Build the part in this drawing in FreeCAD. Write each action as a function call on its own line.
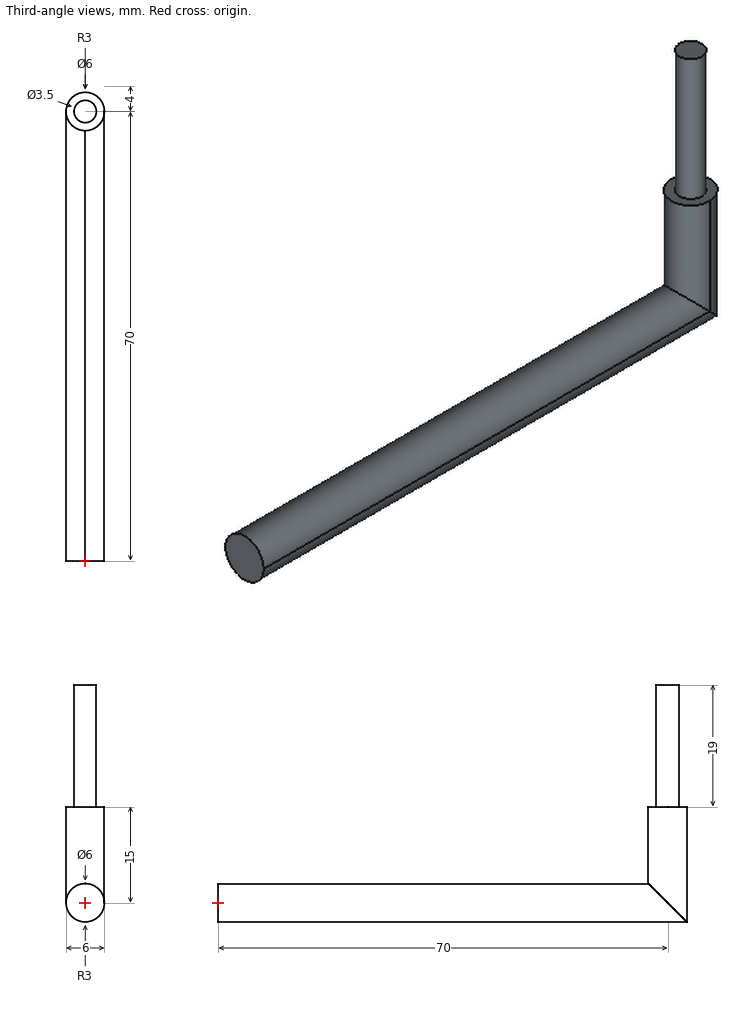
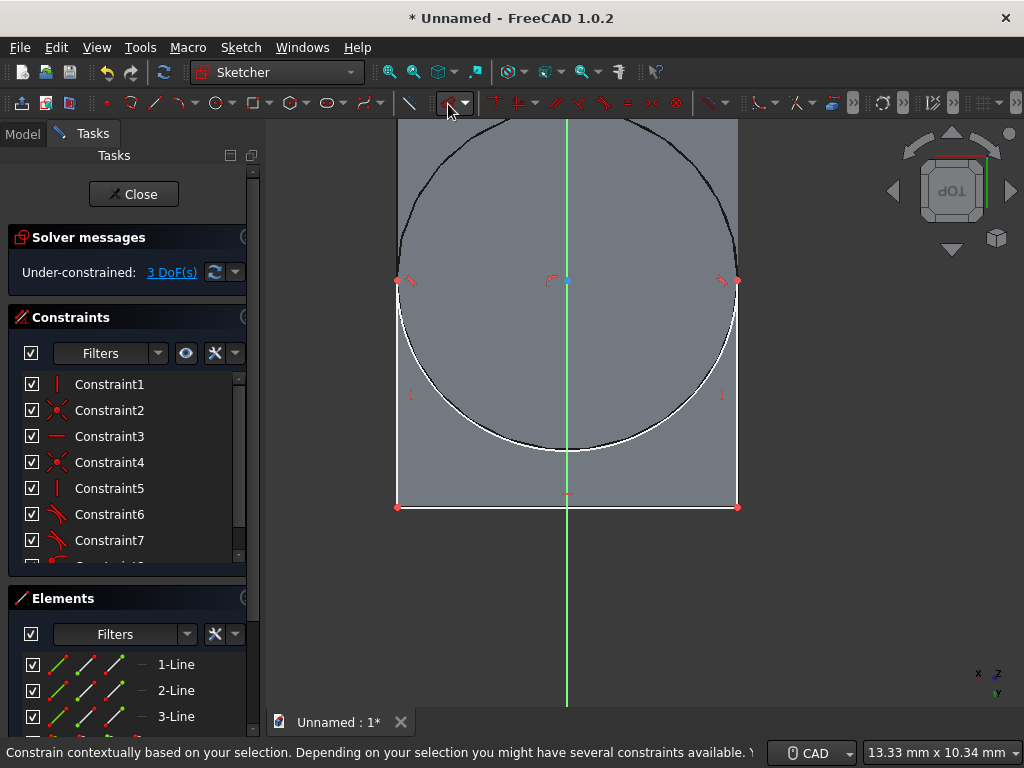
click(467, 419)
click(448, 445)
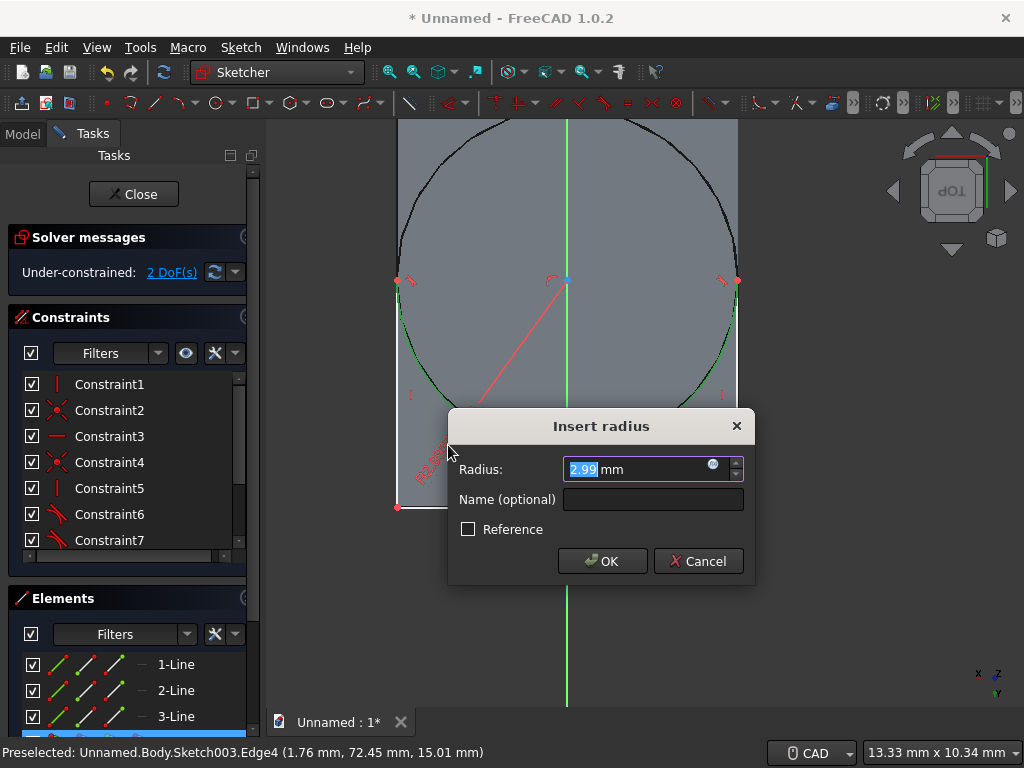
text(3)
key(Return)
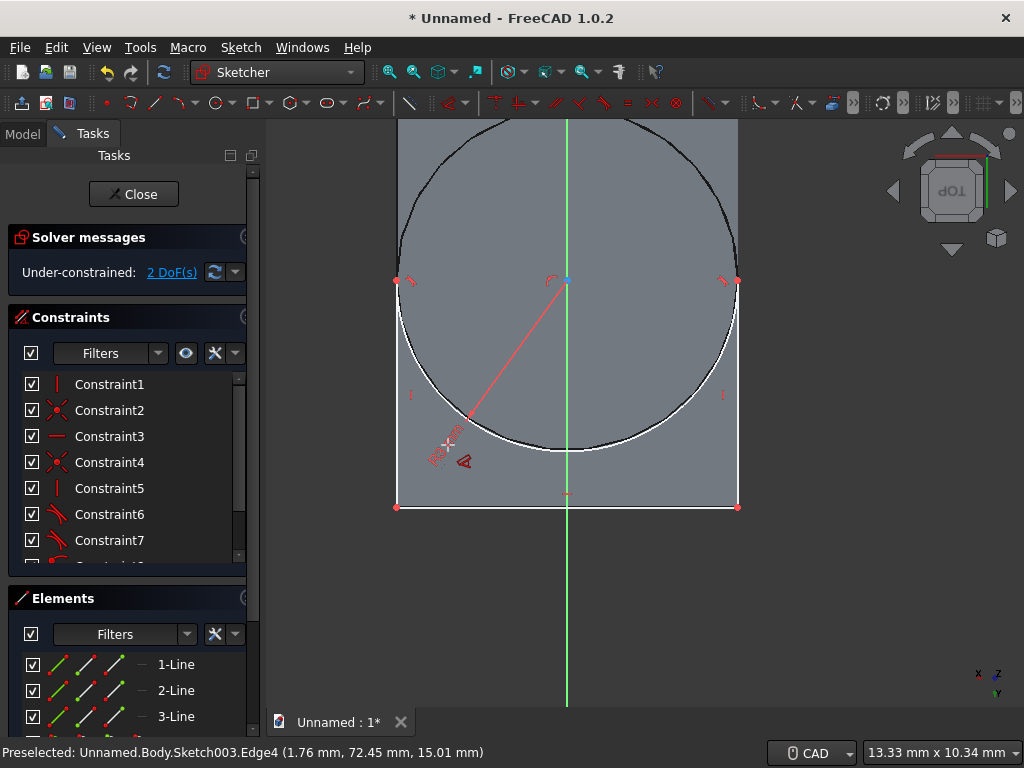
click(397, 349)
click(363, 394)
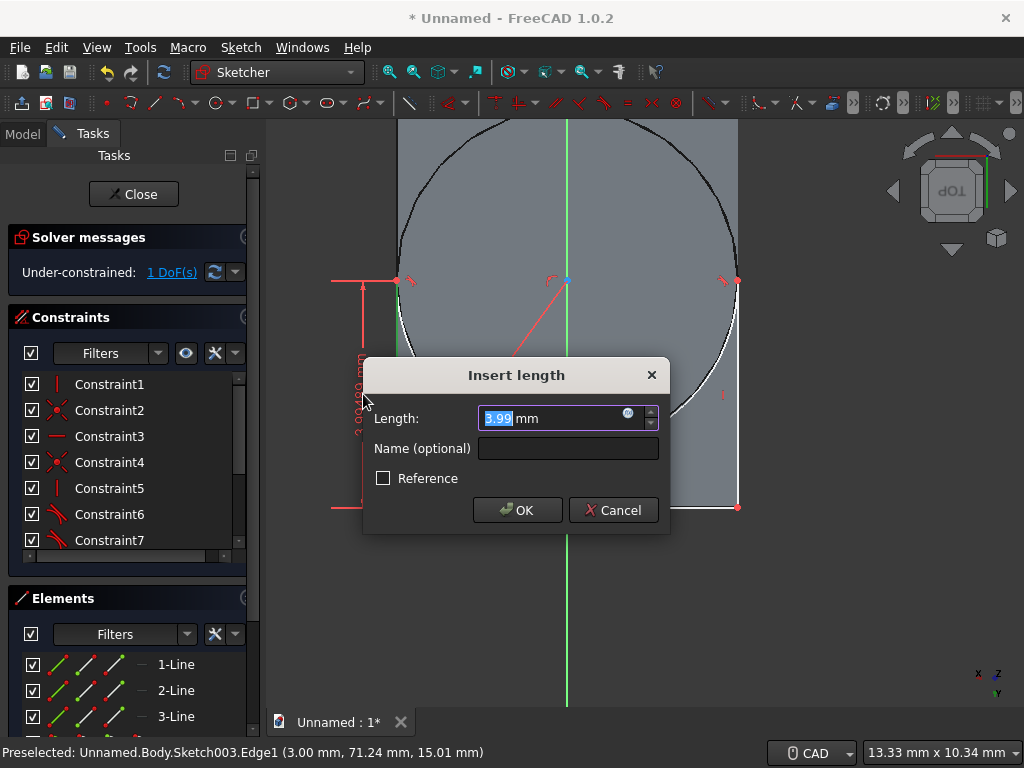
text(4)
key(Return)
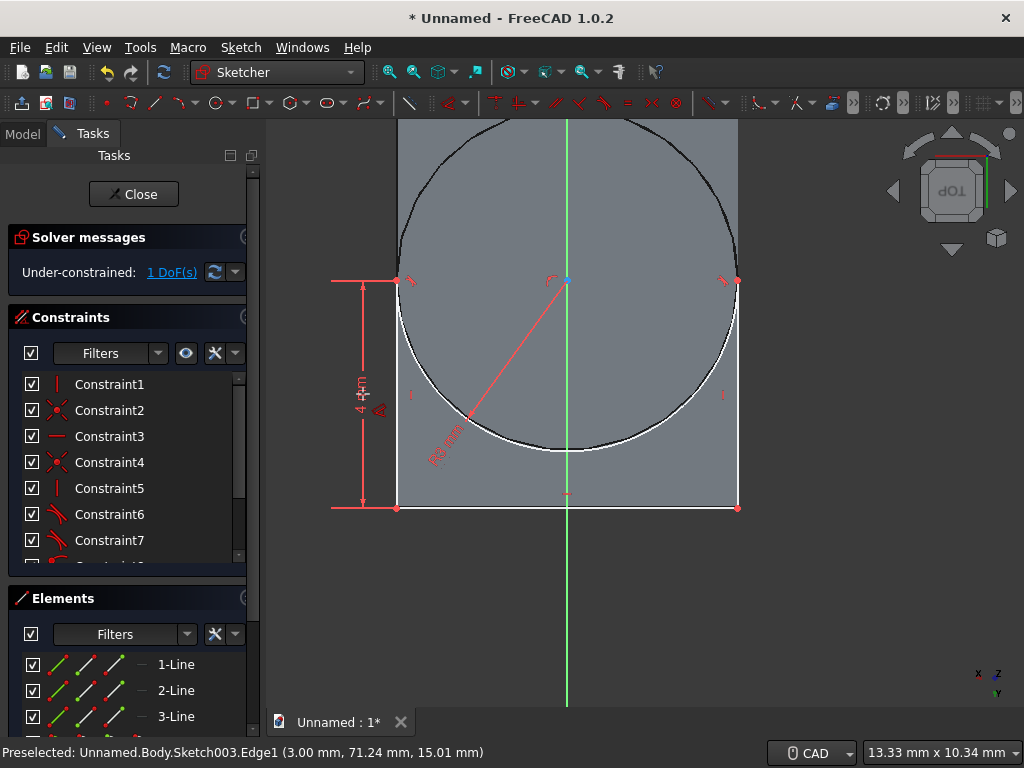
click(397, 281)
click(363, 214)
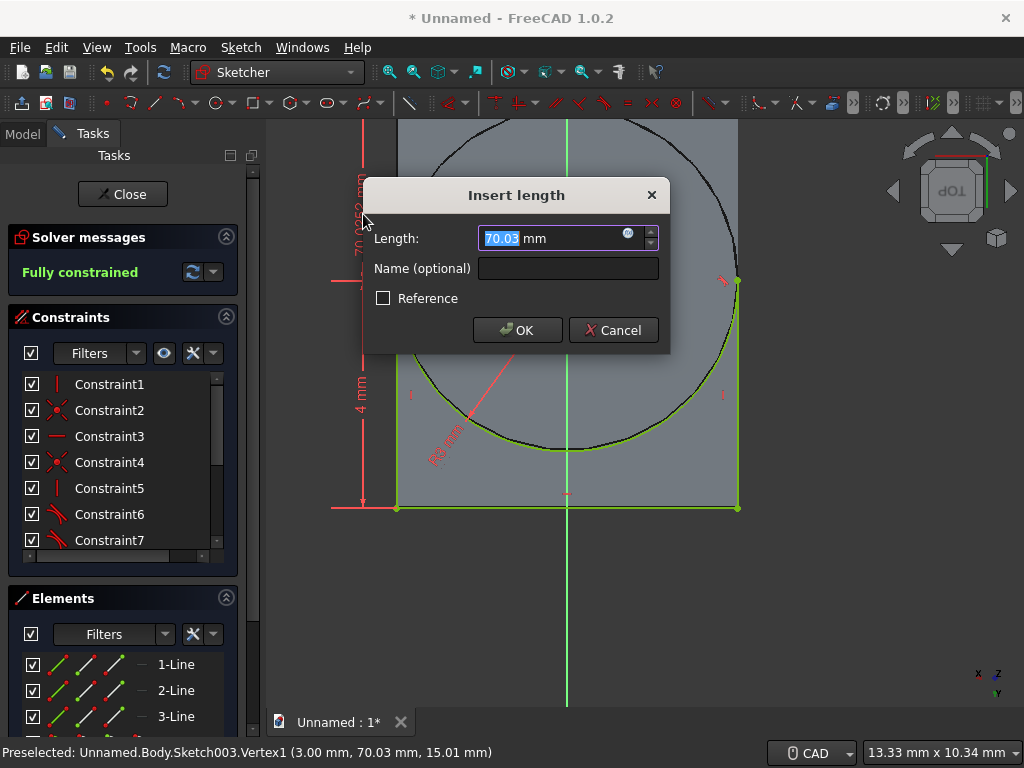
text(70)
key(Return)
key(Escape)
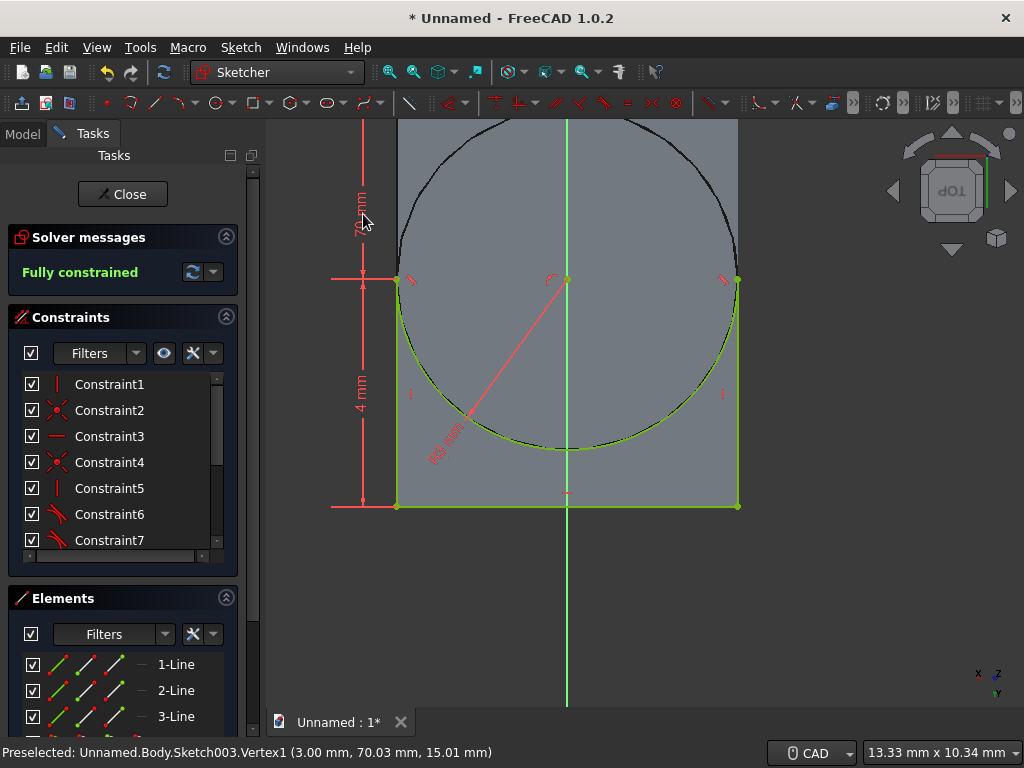
click(123, 194)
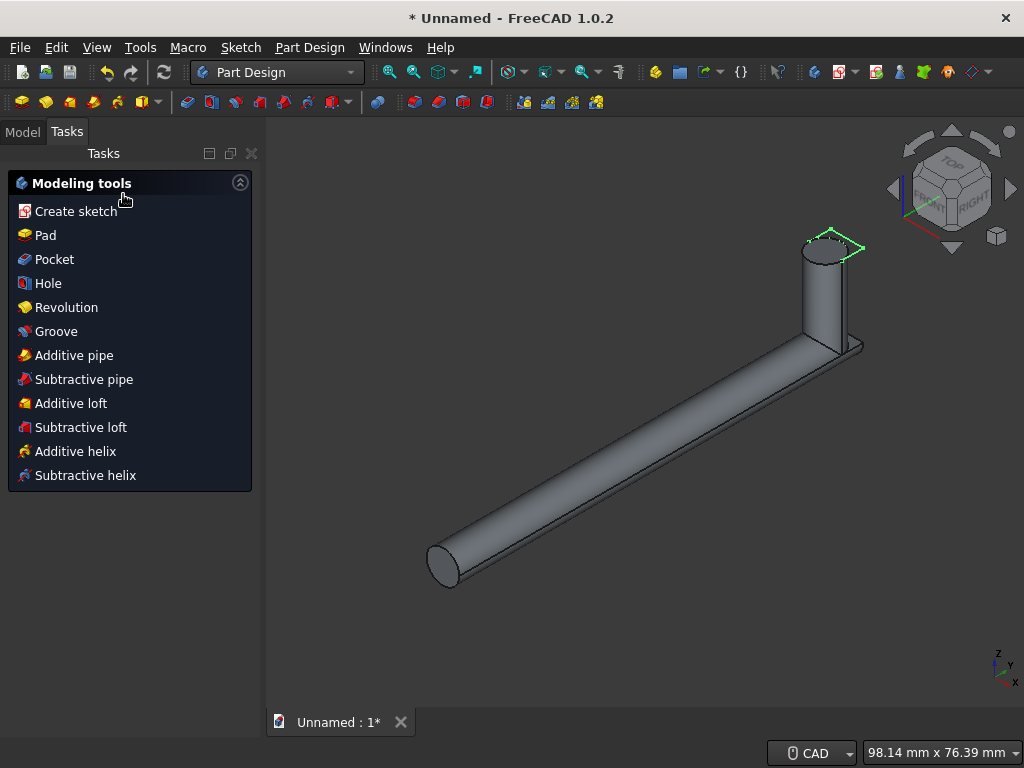
click(188, 102)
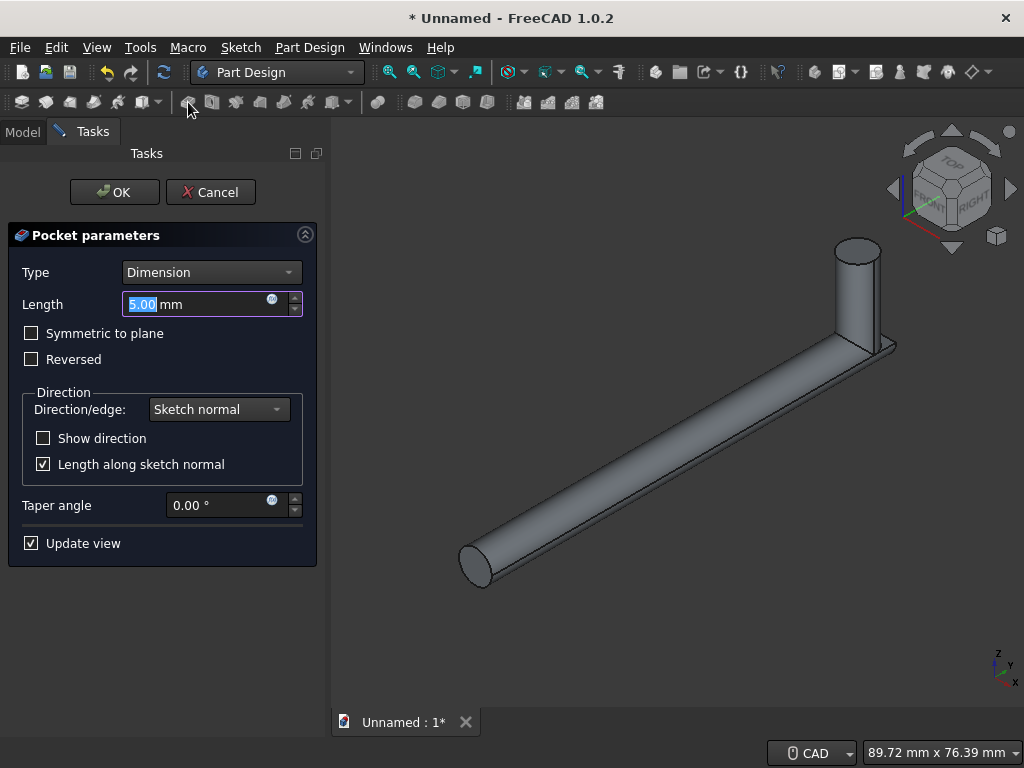
click(212, 272)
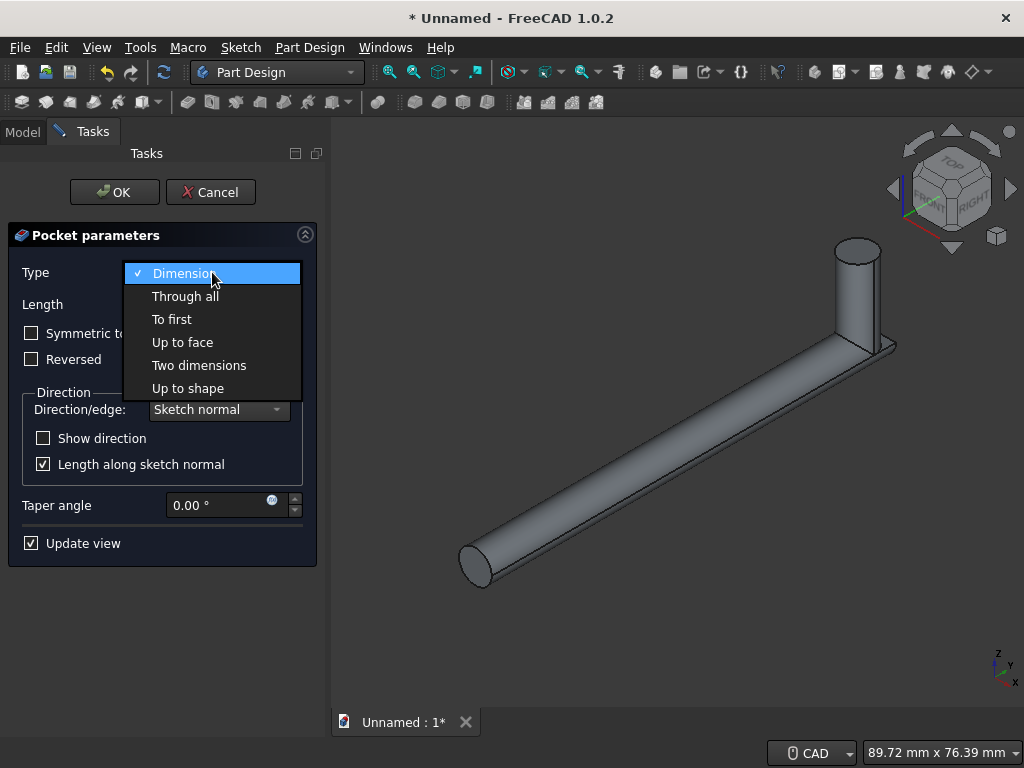
click(212, 296)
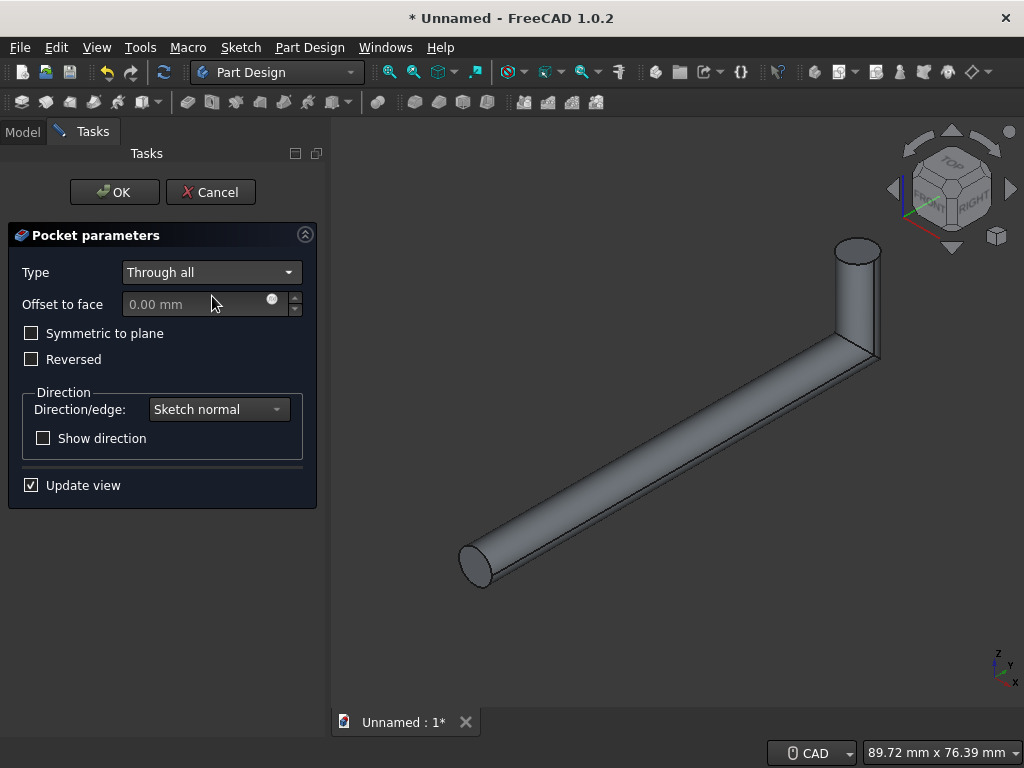
click(115, 192)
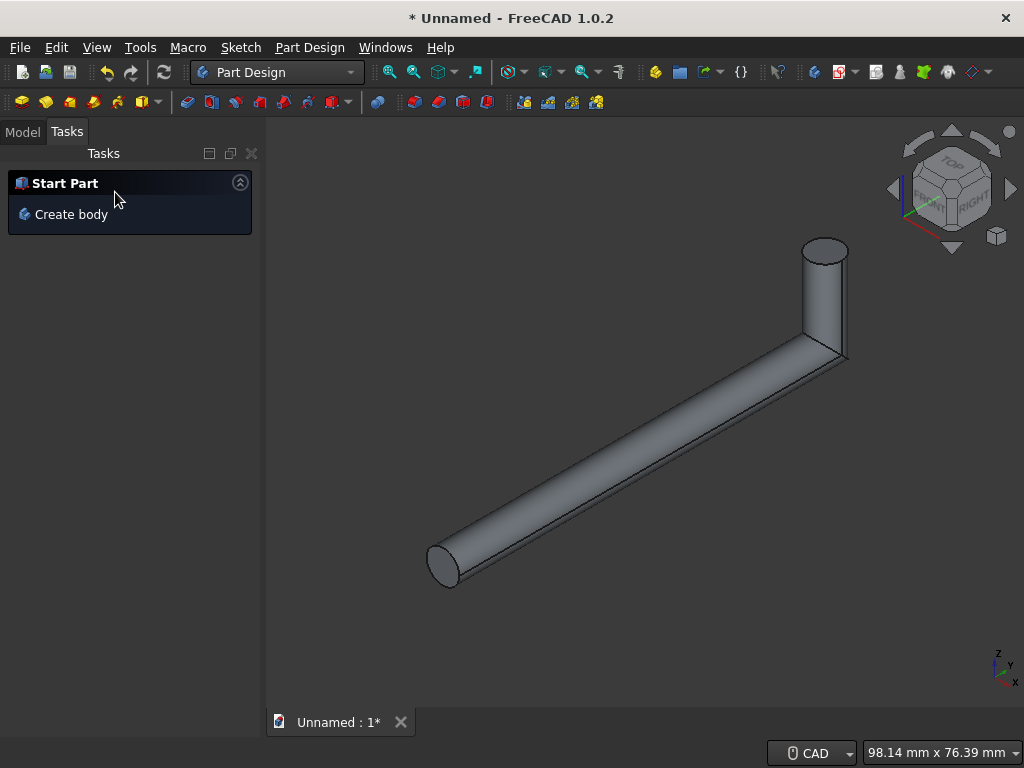
click(825, 250)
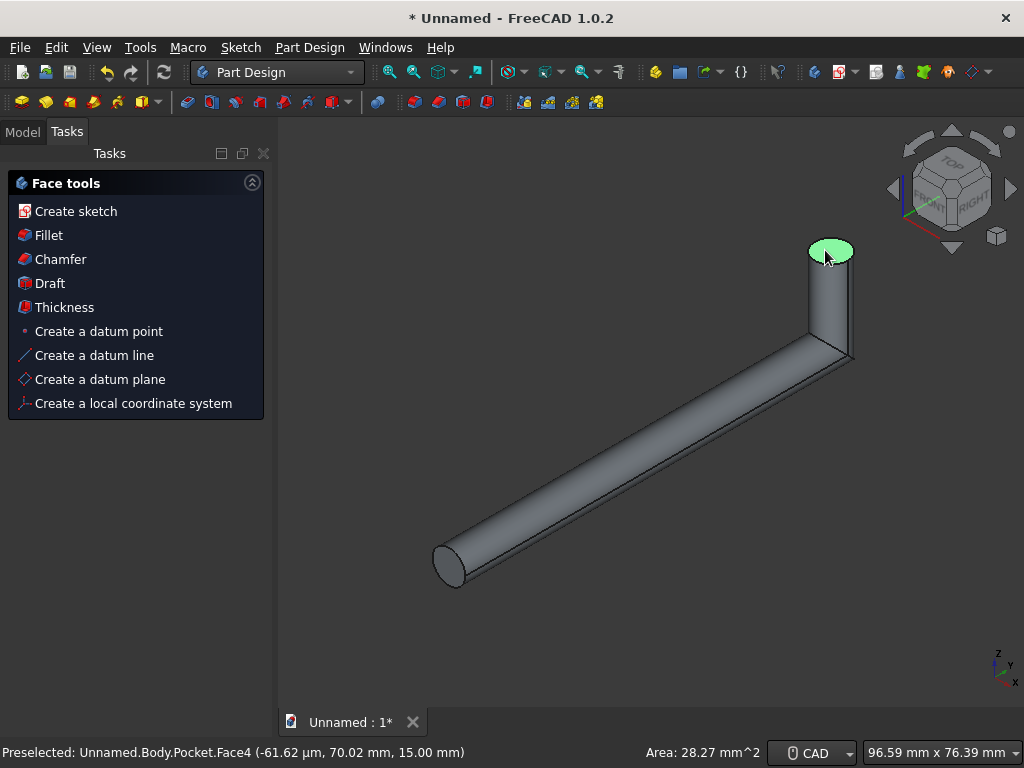
click(840, 72)